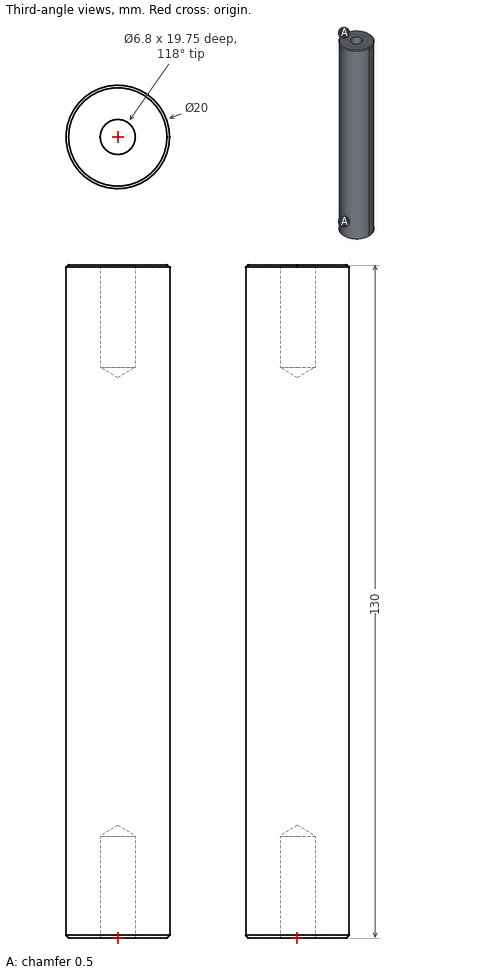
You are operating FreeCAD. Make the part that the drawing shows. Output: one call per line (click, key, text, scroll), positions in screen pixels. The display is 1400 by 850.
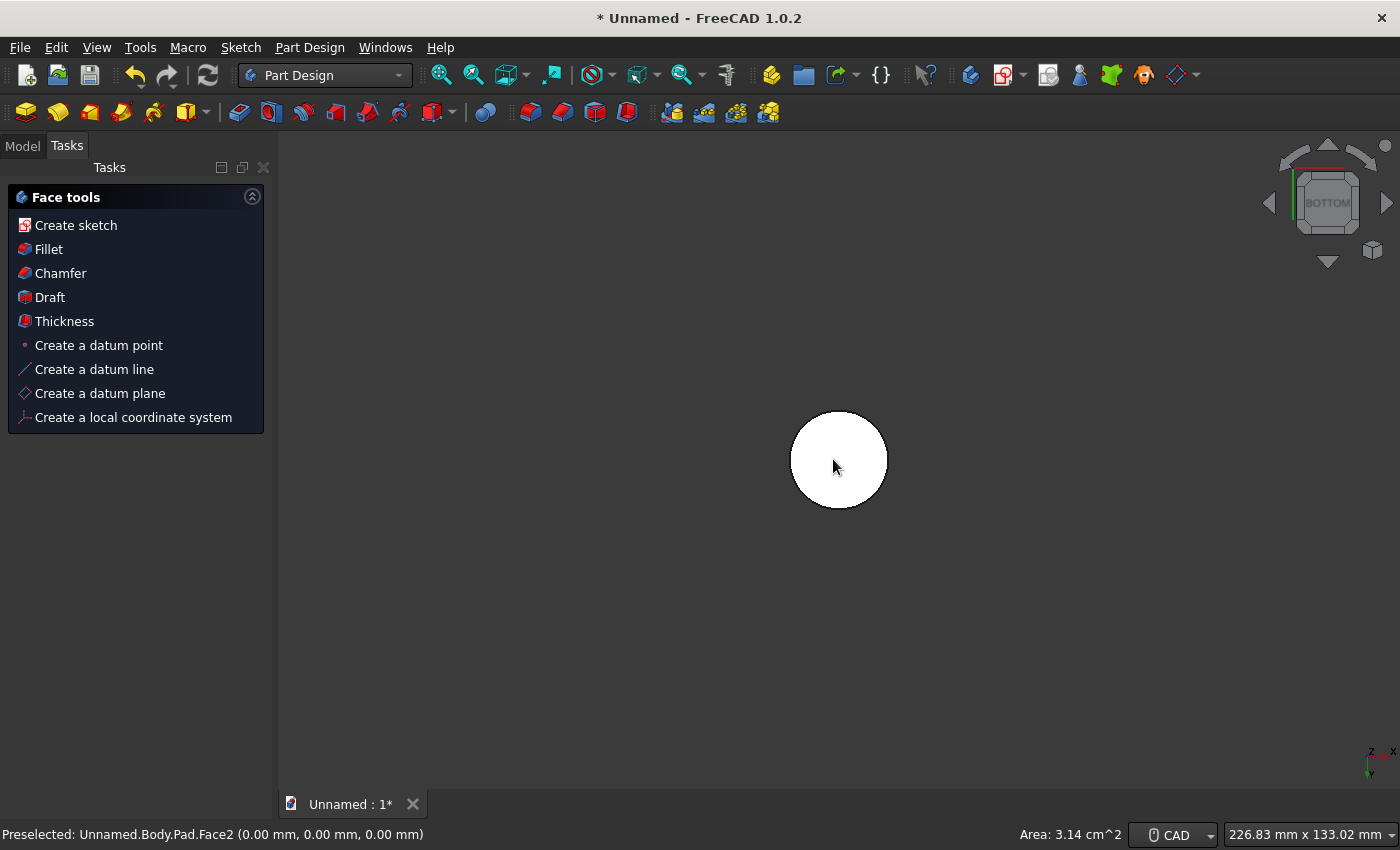
click(1004, 76)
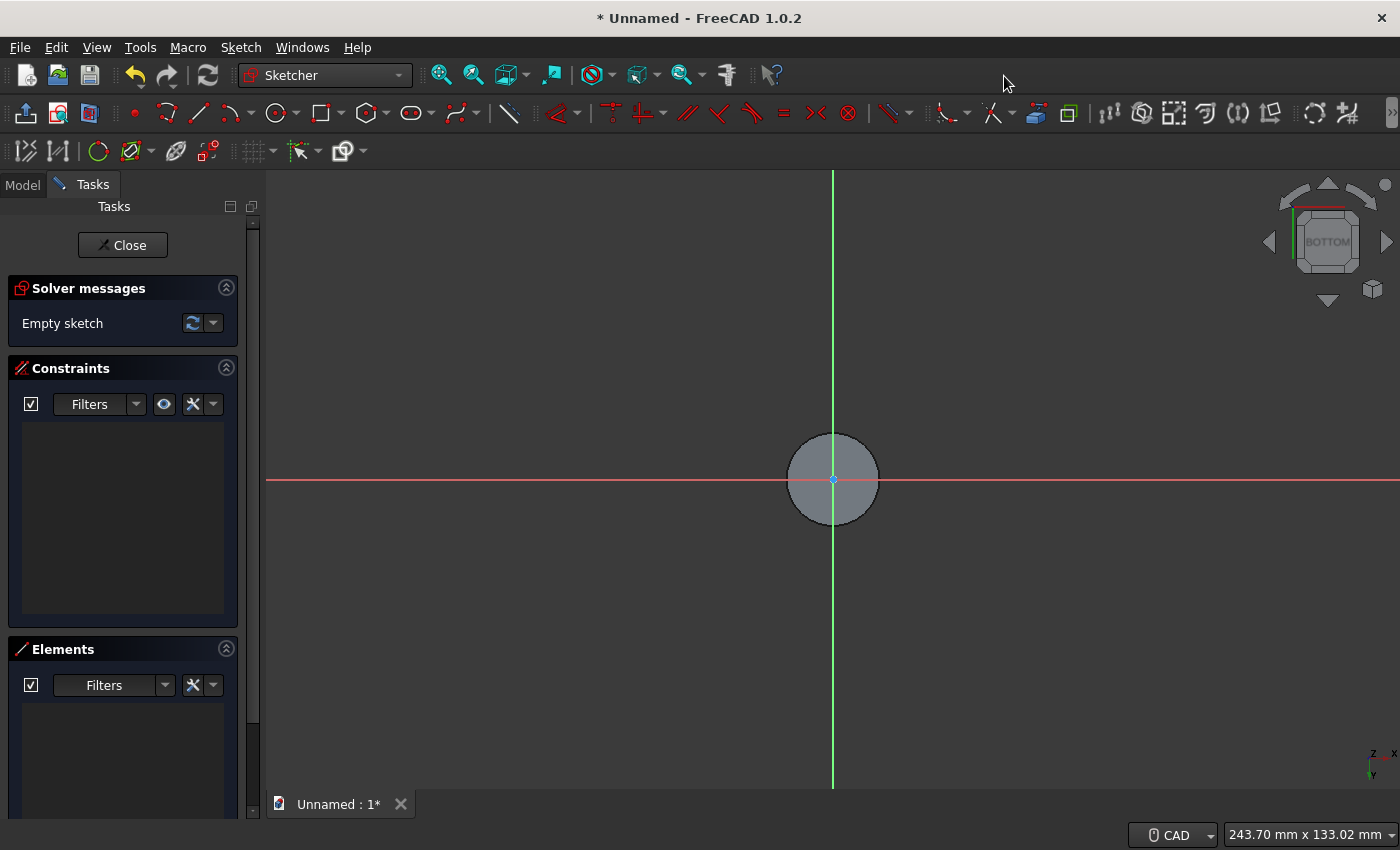
scroll(838, 480, up, 13)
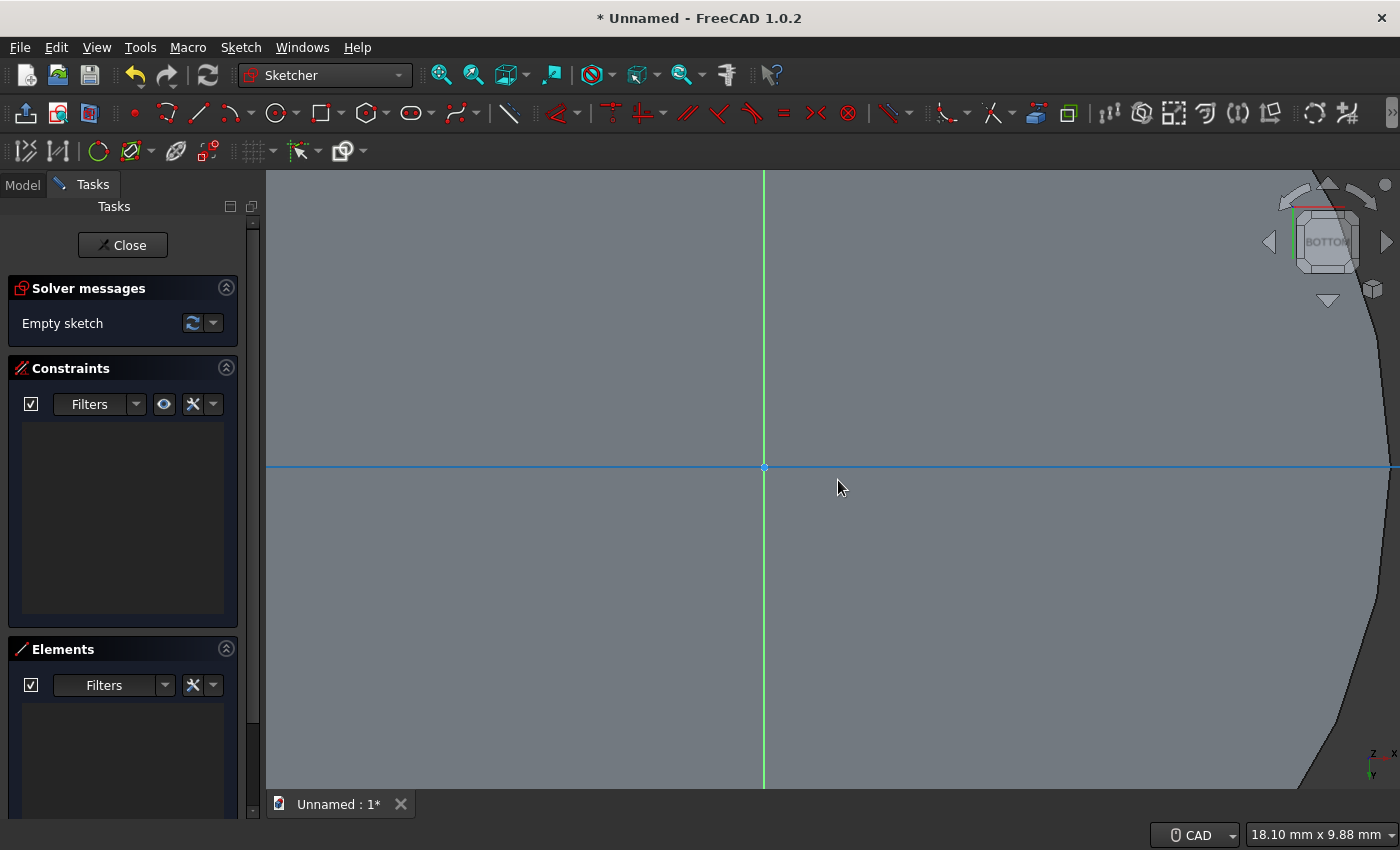
key(g)
key(c)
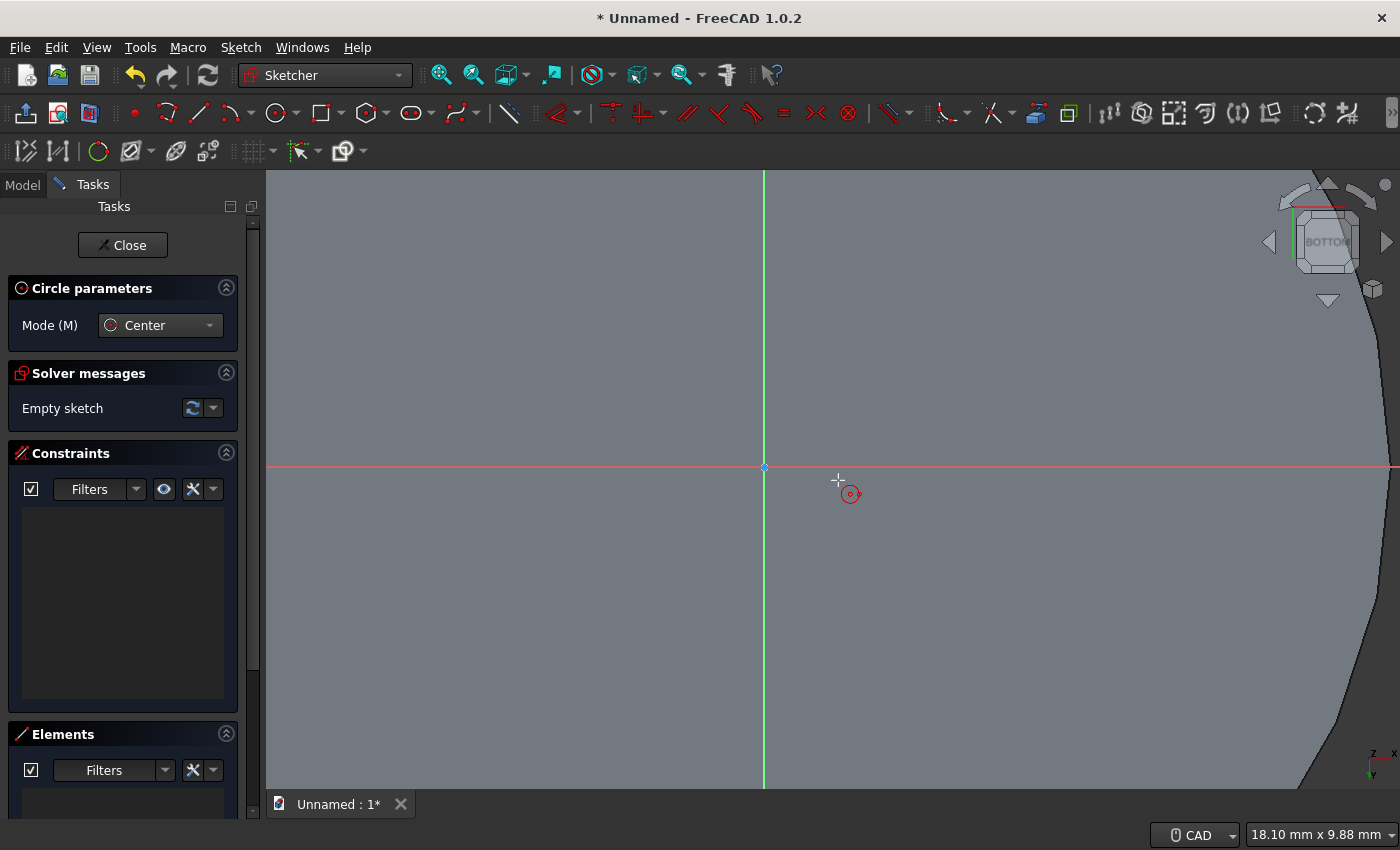
click(764, 467)
click(915, 316)
key(Escape)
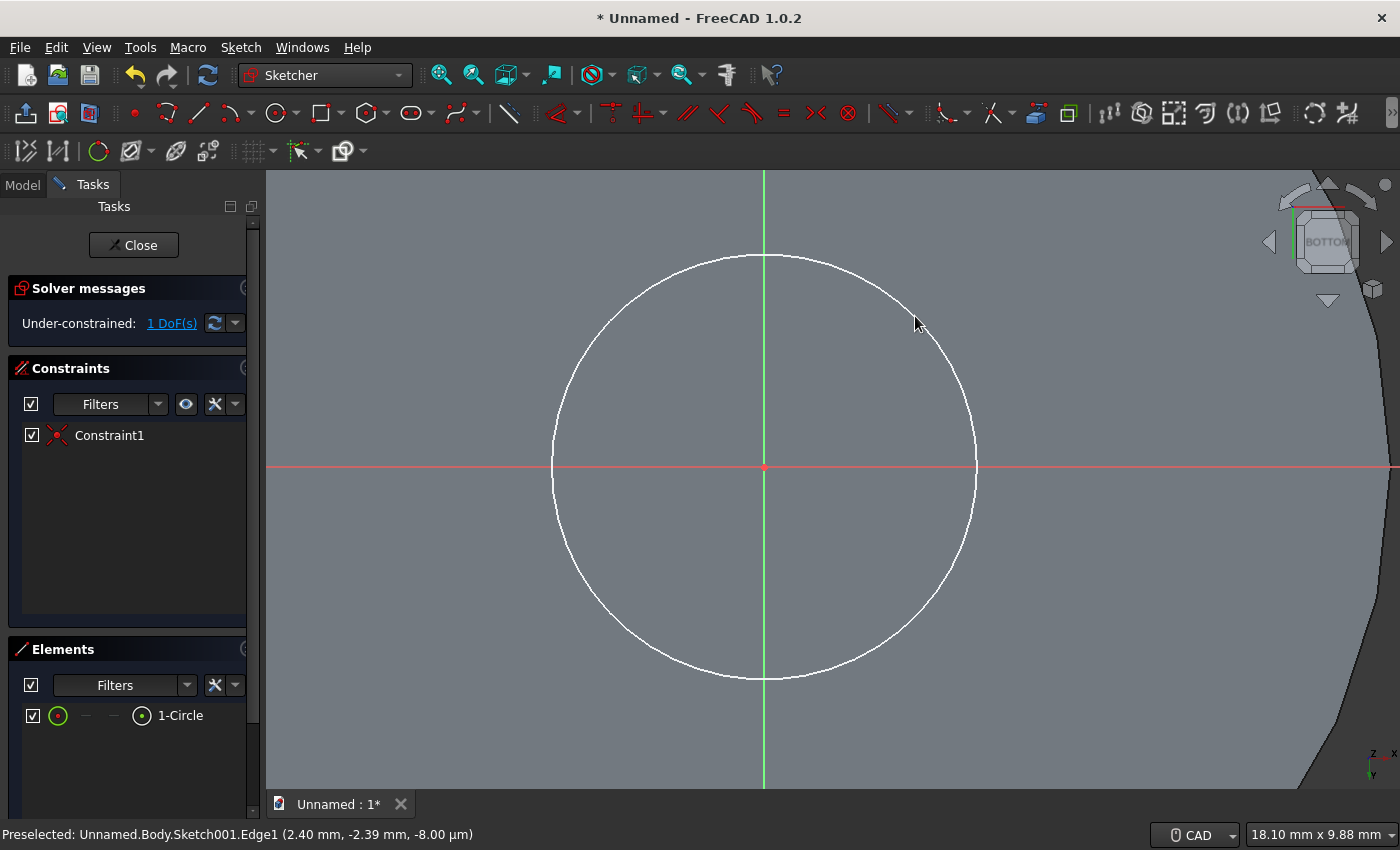
click(556, 114)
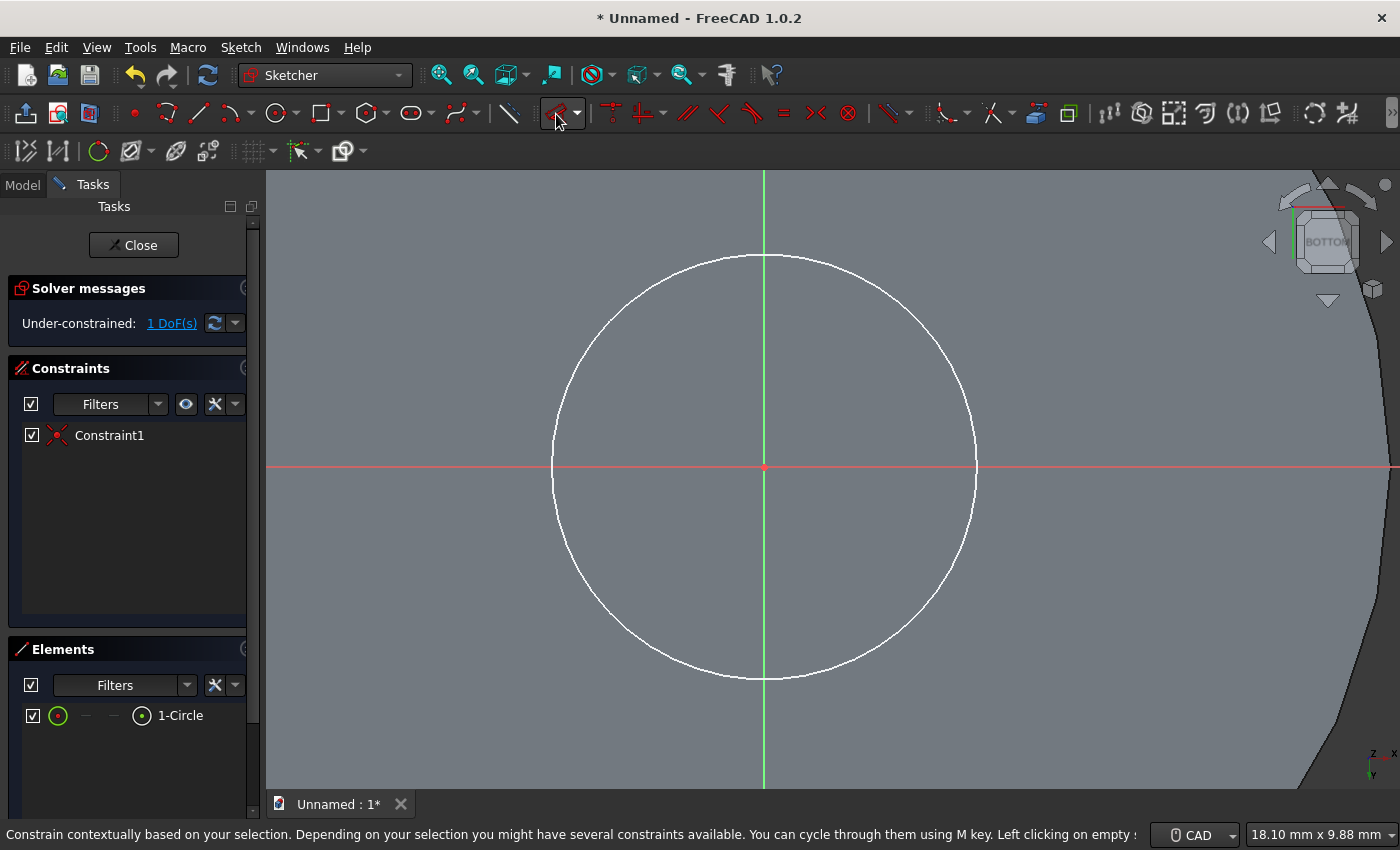
click(914, 316)
click(937, 293)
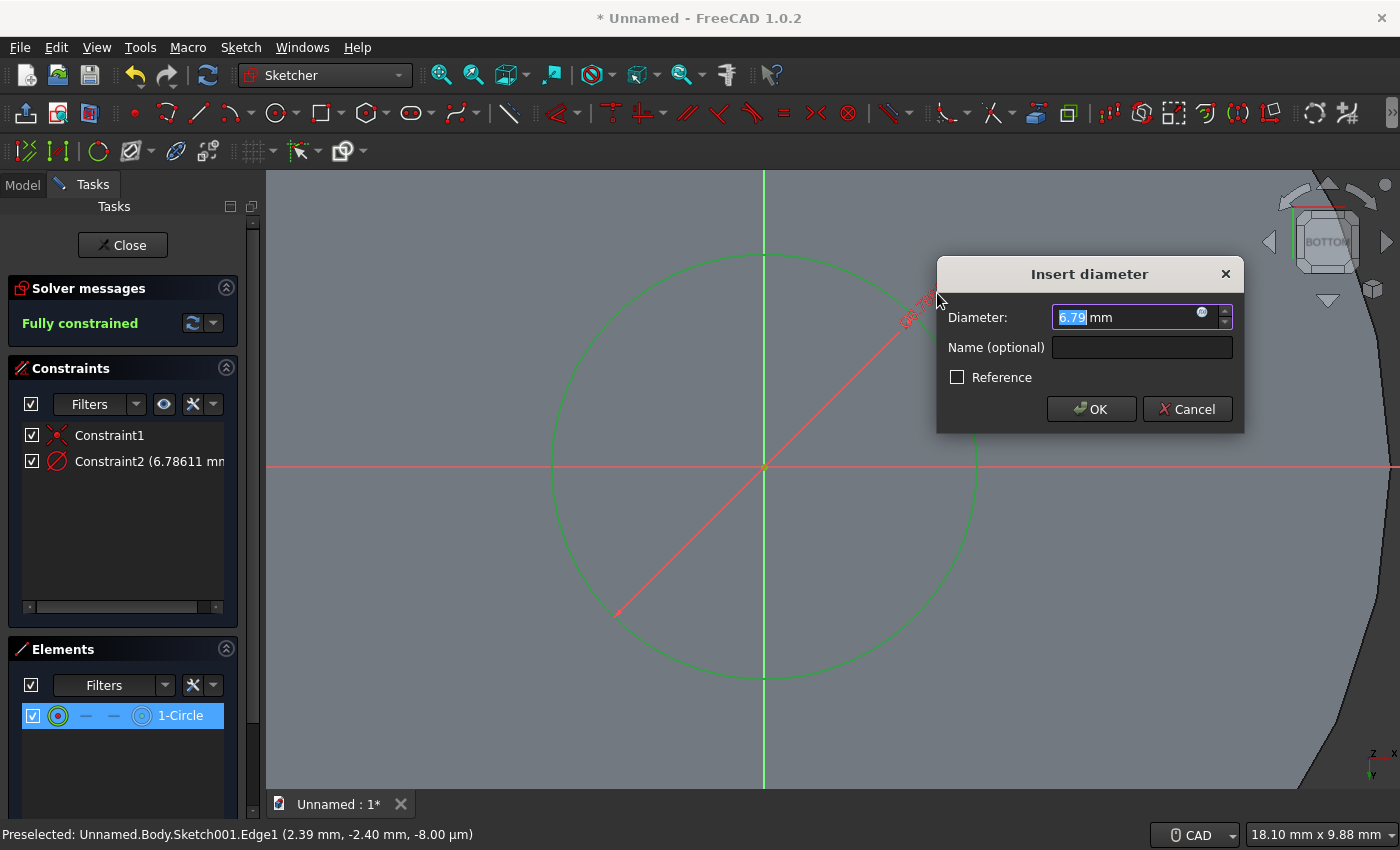
text(6.8)
key(Return)
key(Escape)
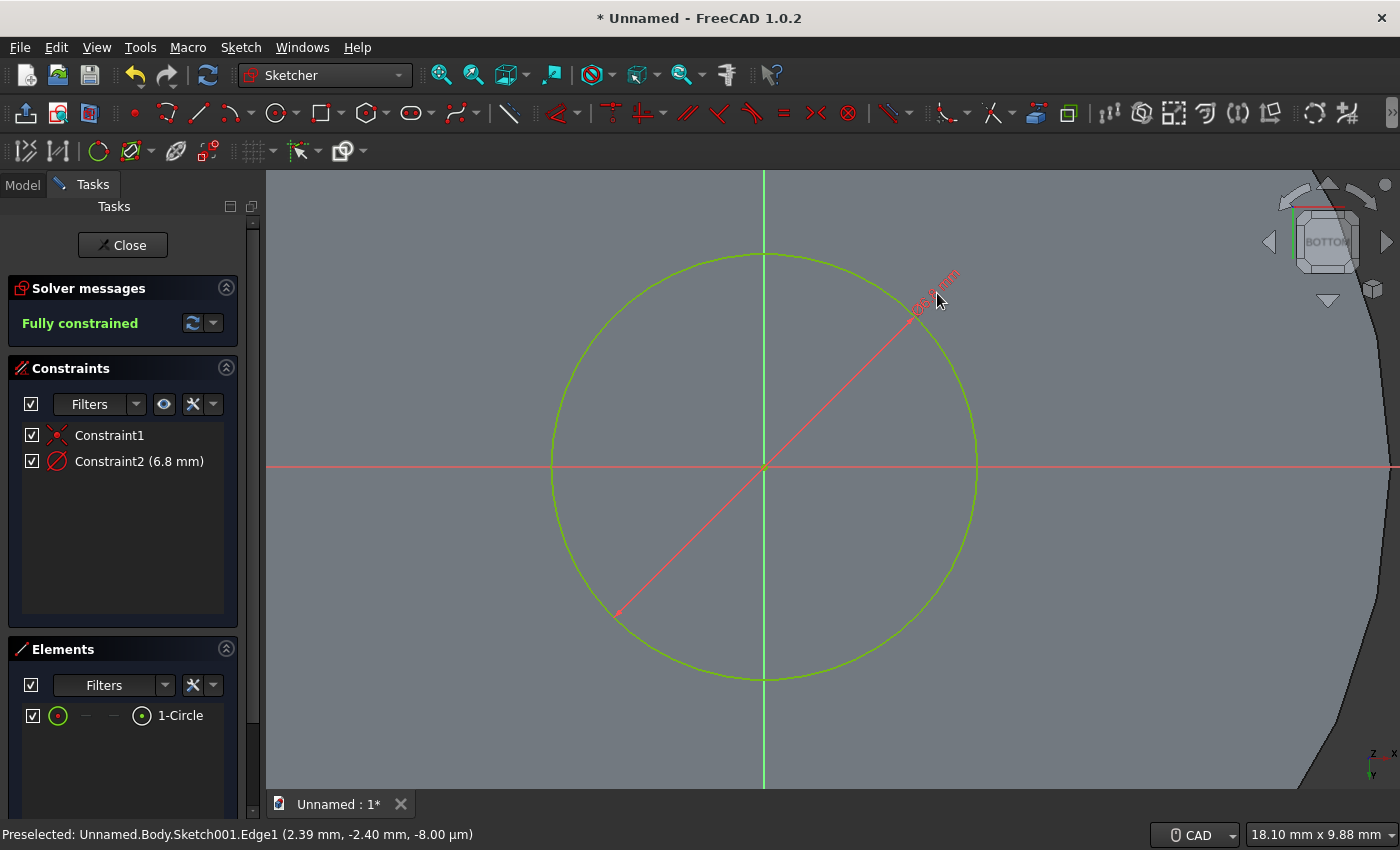
click(123, 245)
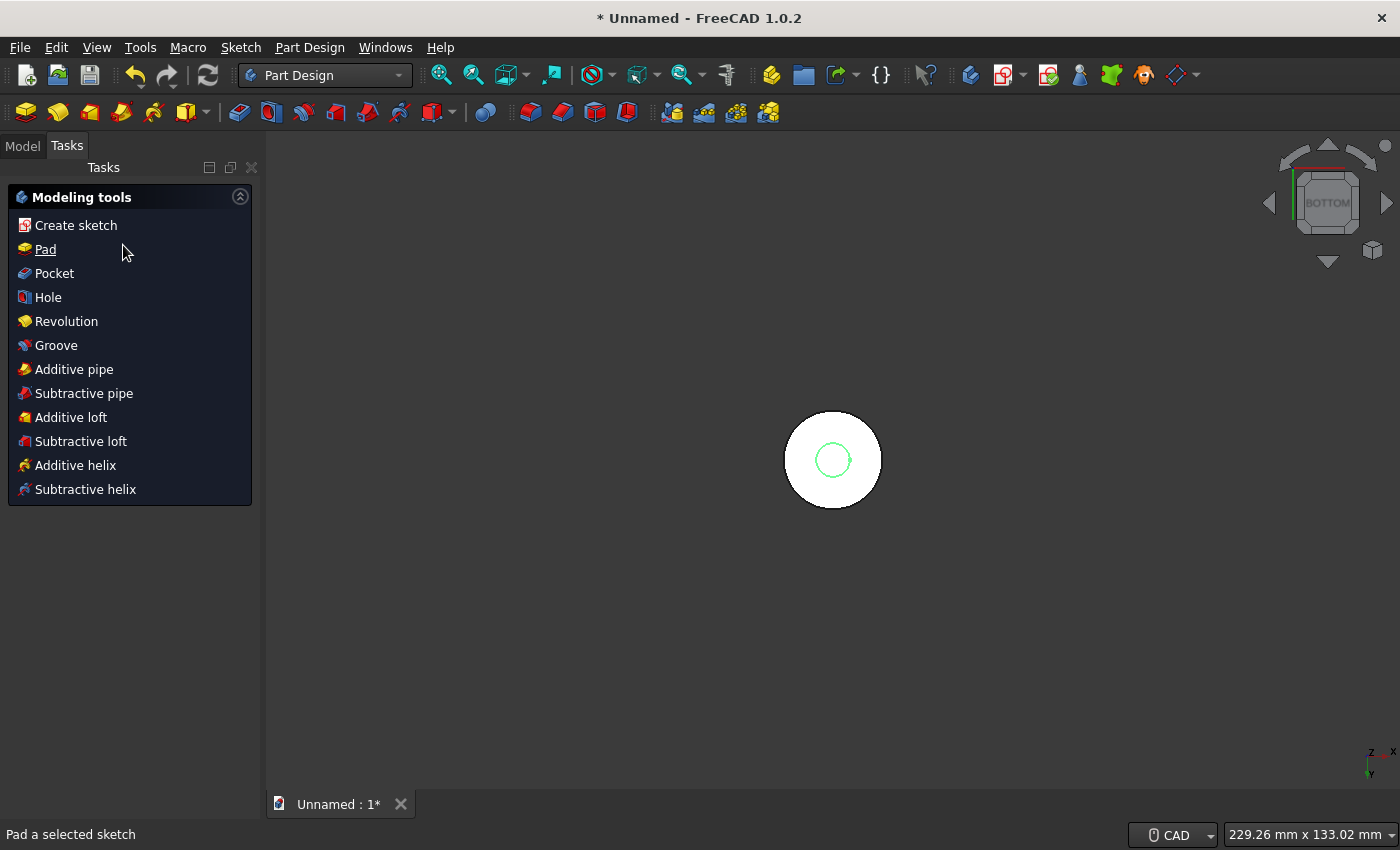
click(272, 112)